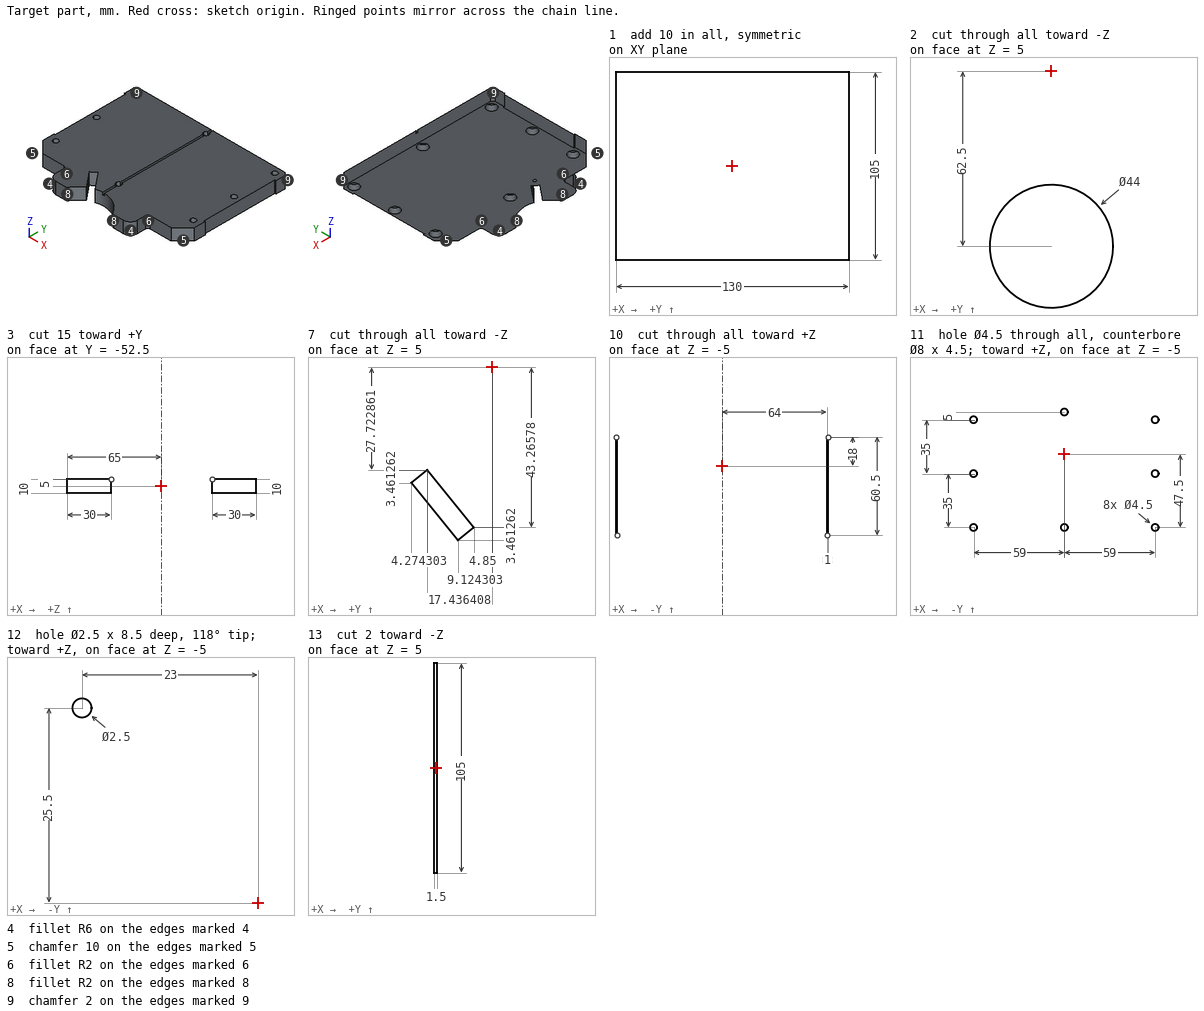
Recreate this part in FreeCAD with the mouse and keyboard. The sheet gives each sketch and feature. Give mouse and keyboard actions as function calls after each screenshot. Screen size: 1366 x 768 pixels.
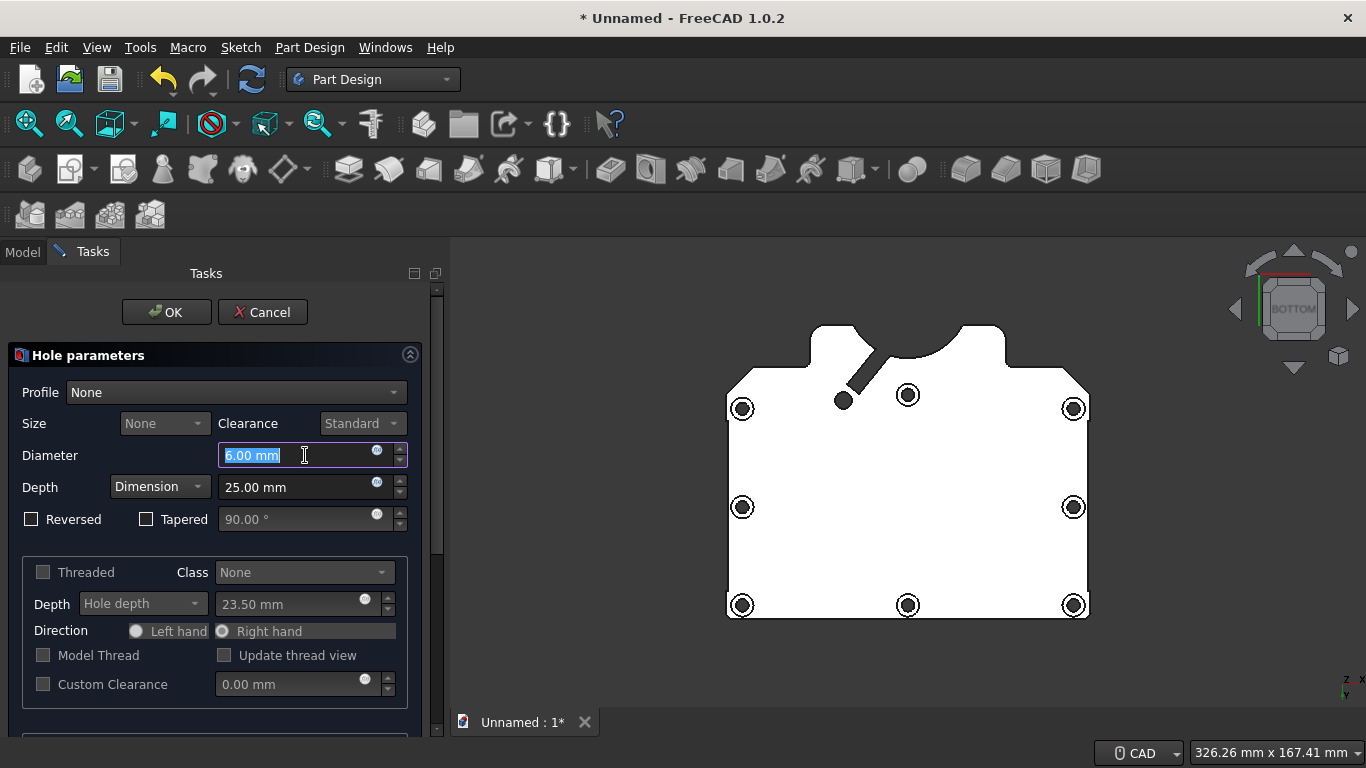
text(2.5)
key(Tab)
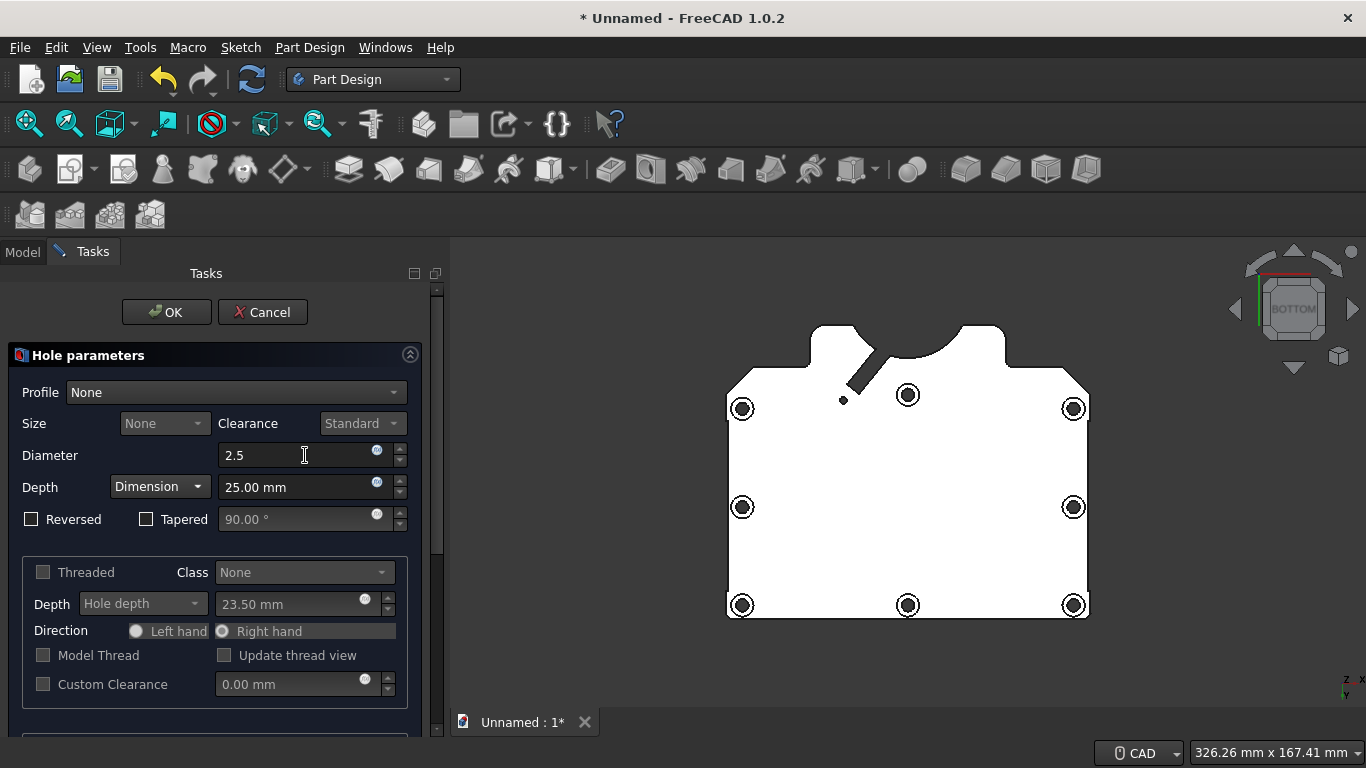
triple_click(305, 487)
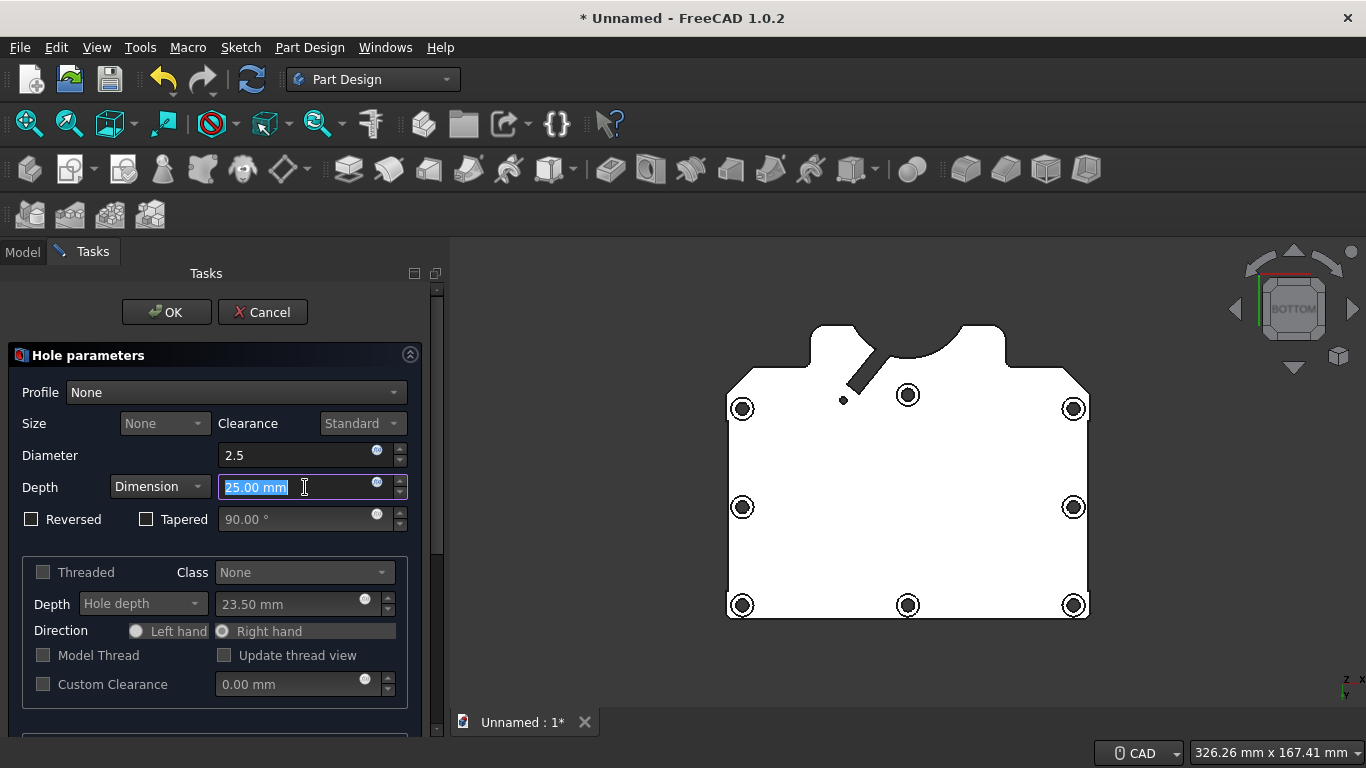
text(8.5)
key(Tab)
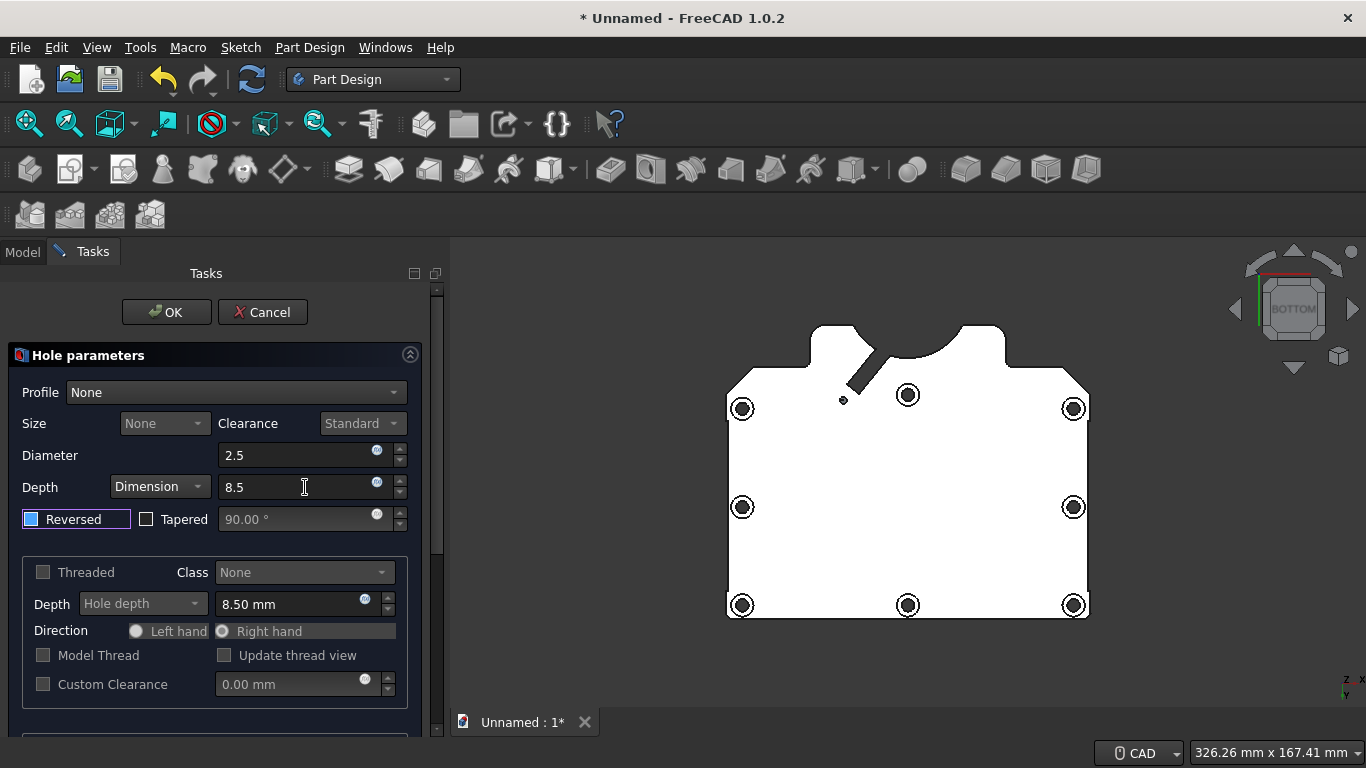
click(167, 312)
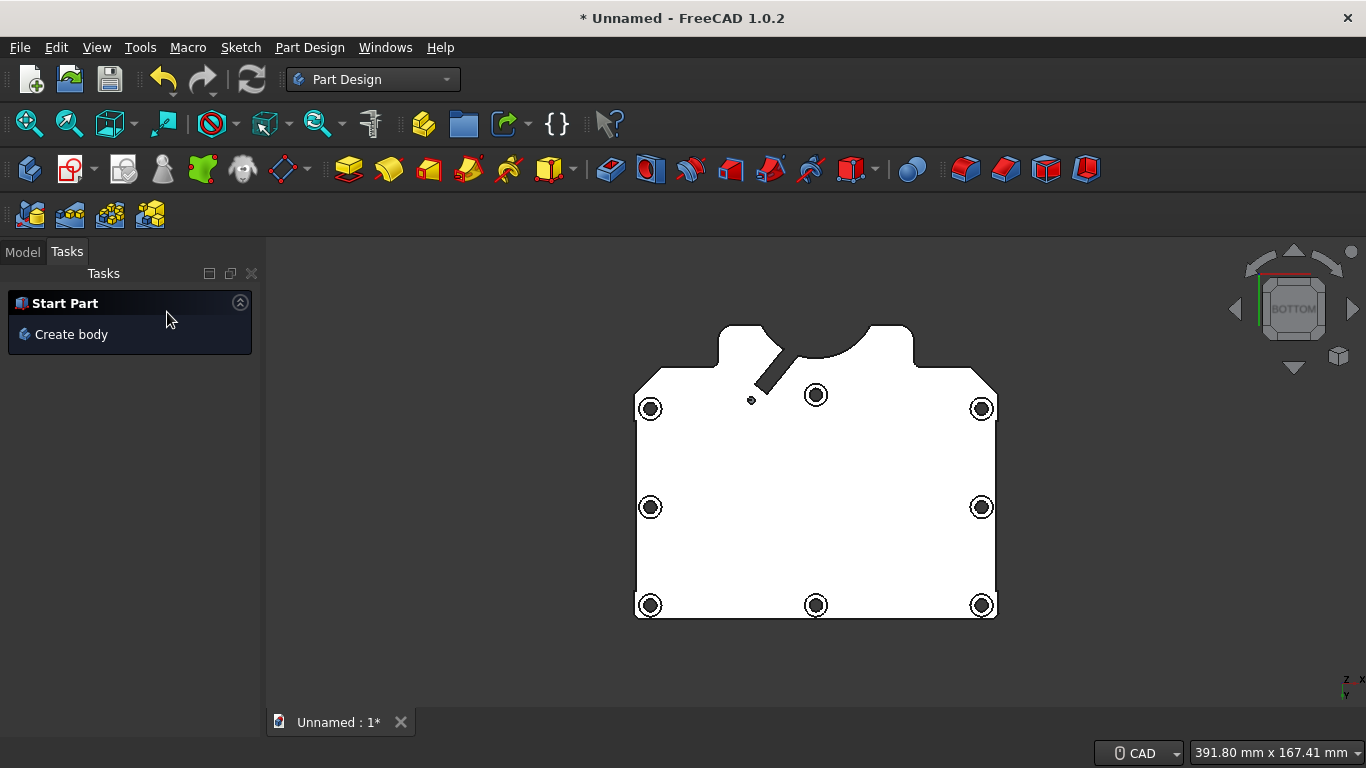
key(0)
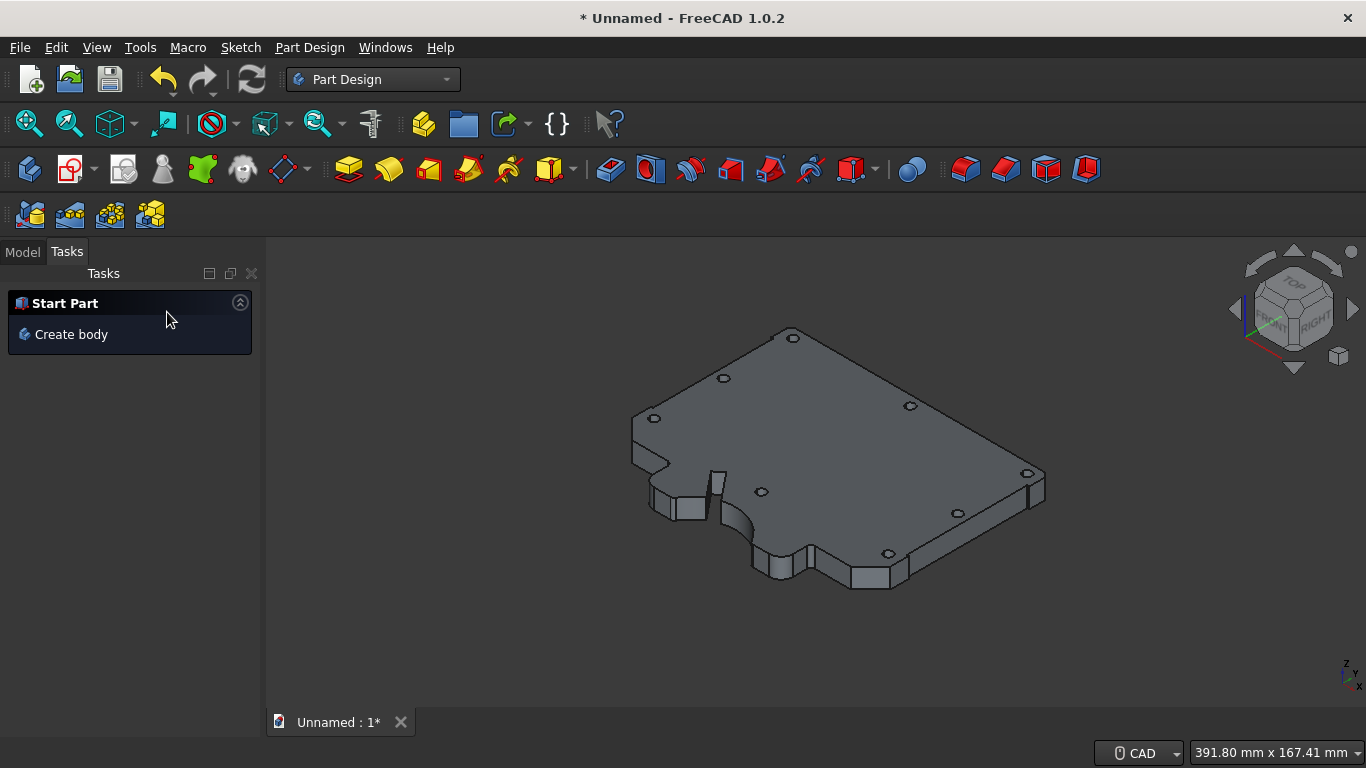
click(883, 464)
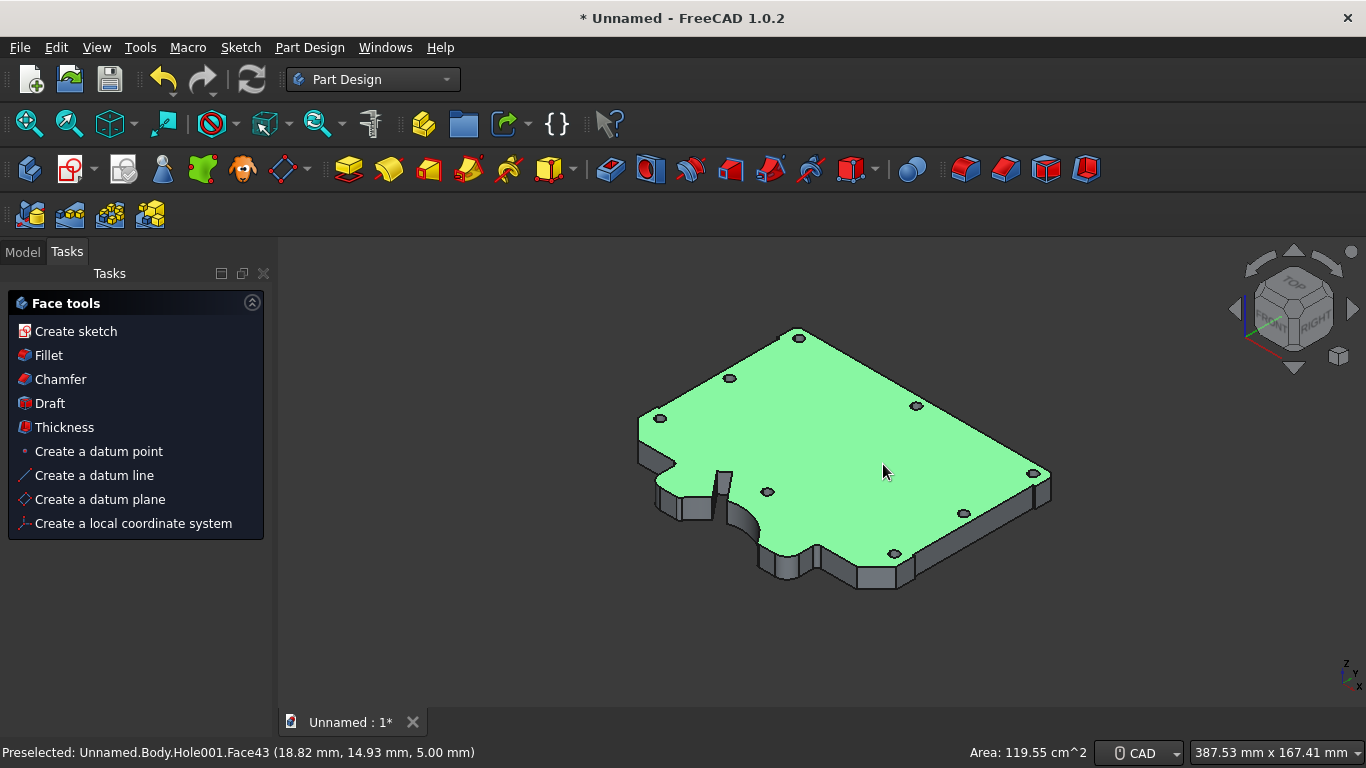
click(70, 170)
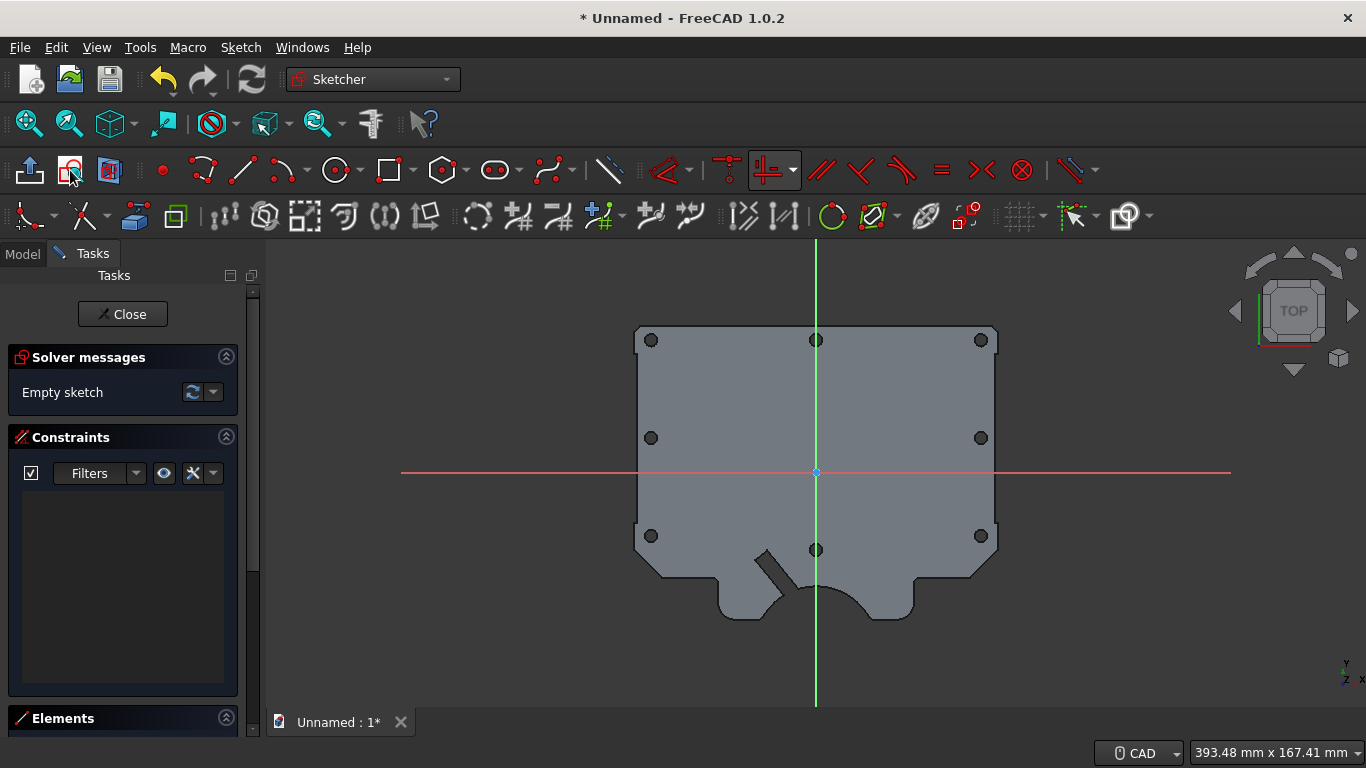
click(416, 170)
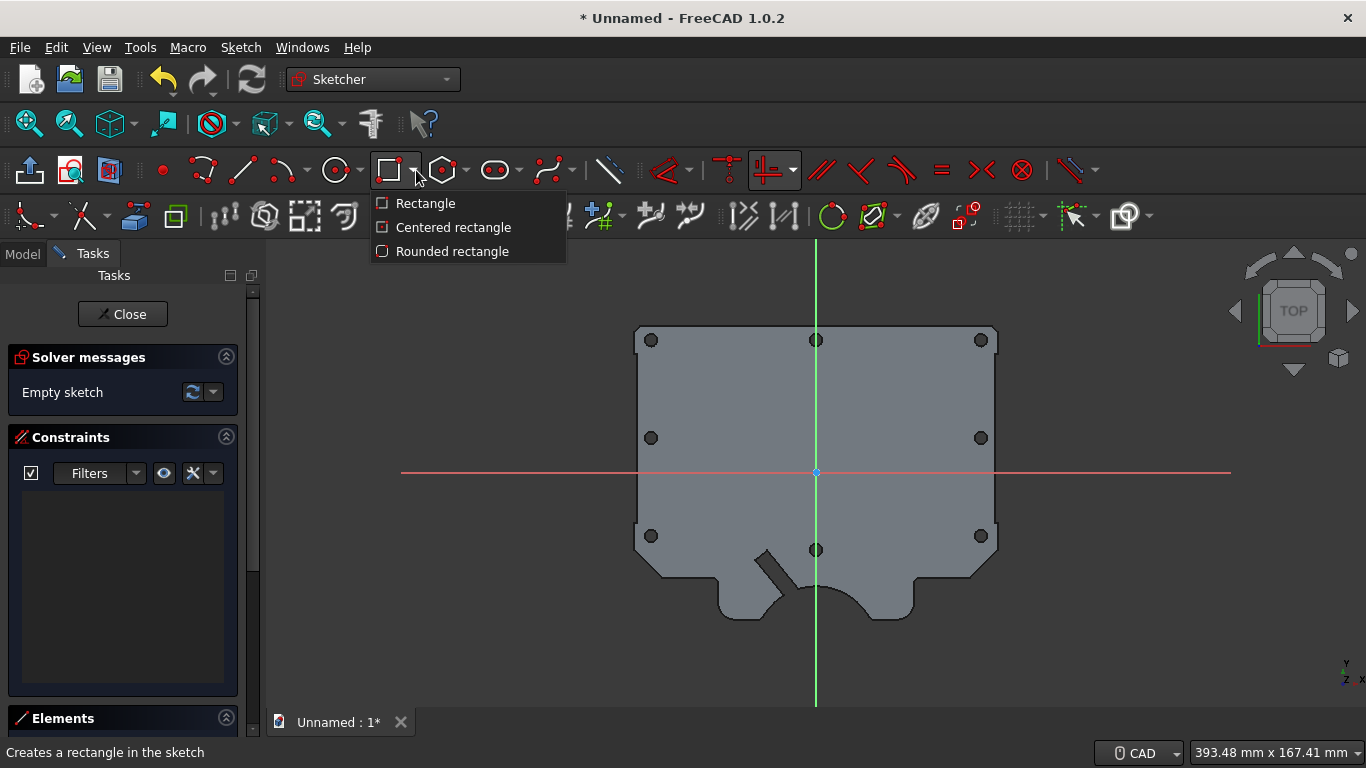
click(468, 227)